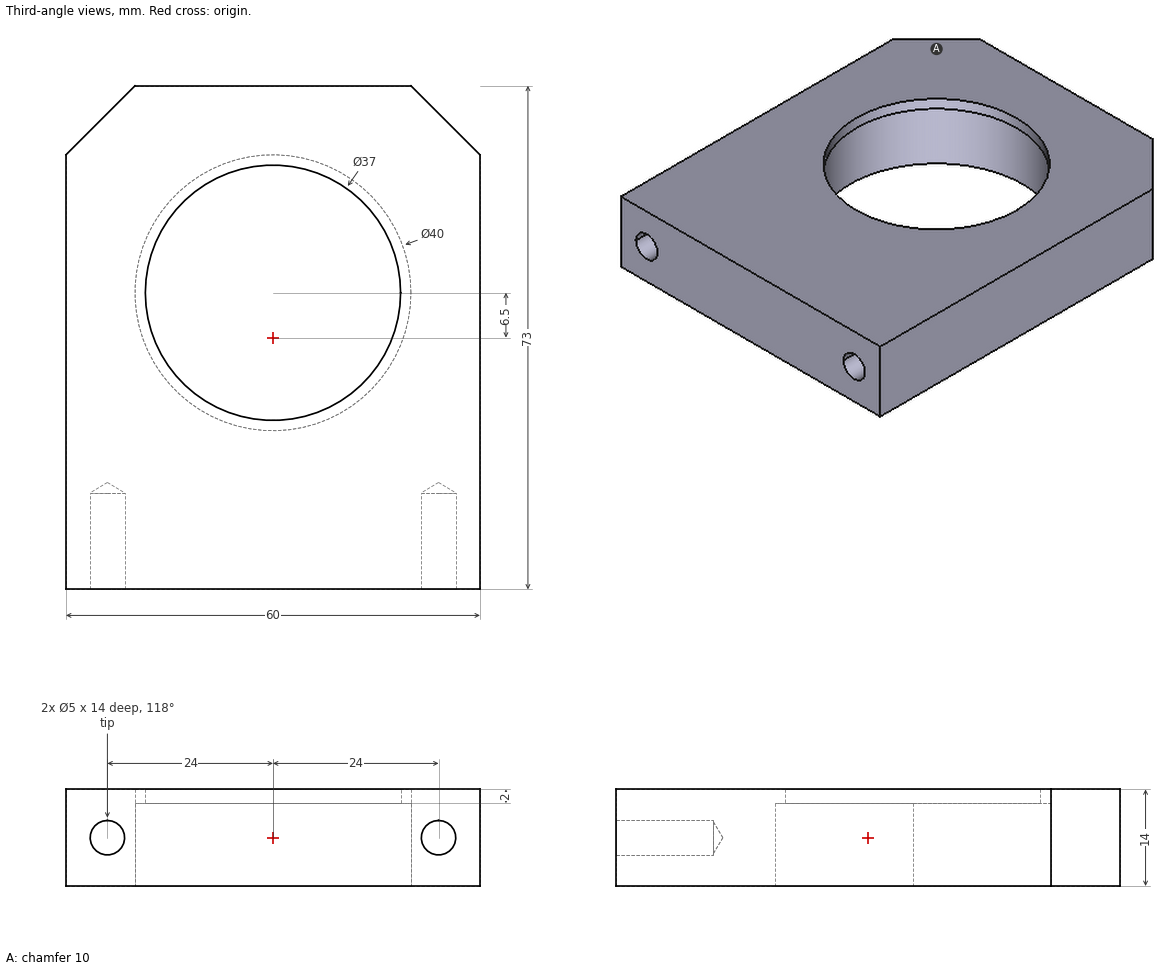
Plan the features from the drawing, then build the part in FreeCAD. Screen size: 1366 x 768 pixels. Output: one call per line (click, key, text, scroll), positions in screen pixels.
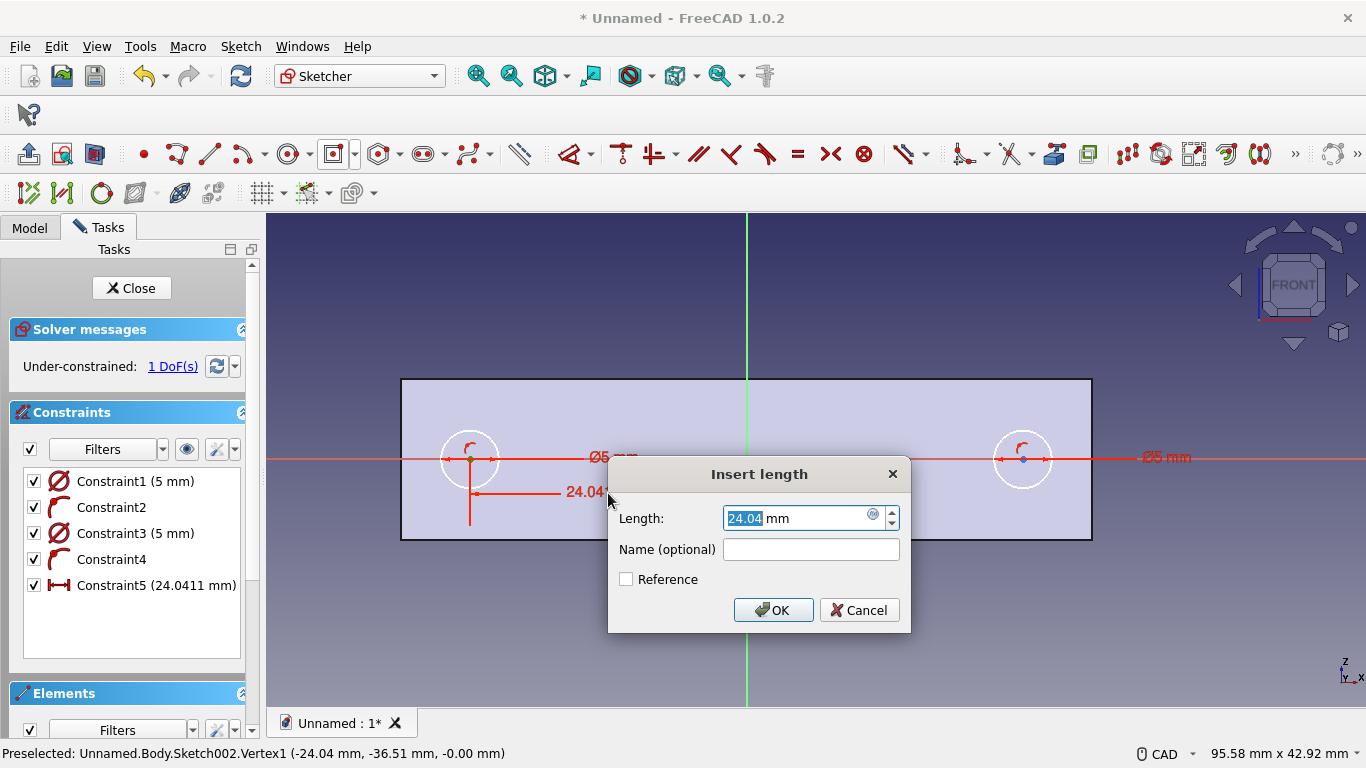
text(24)
key(Return)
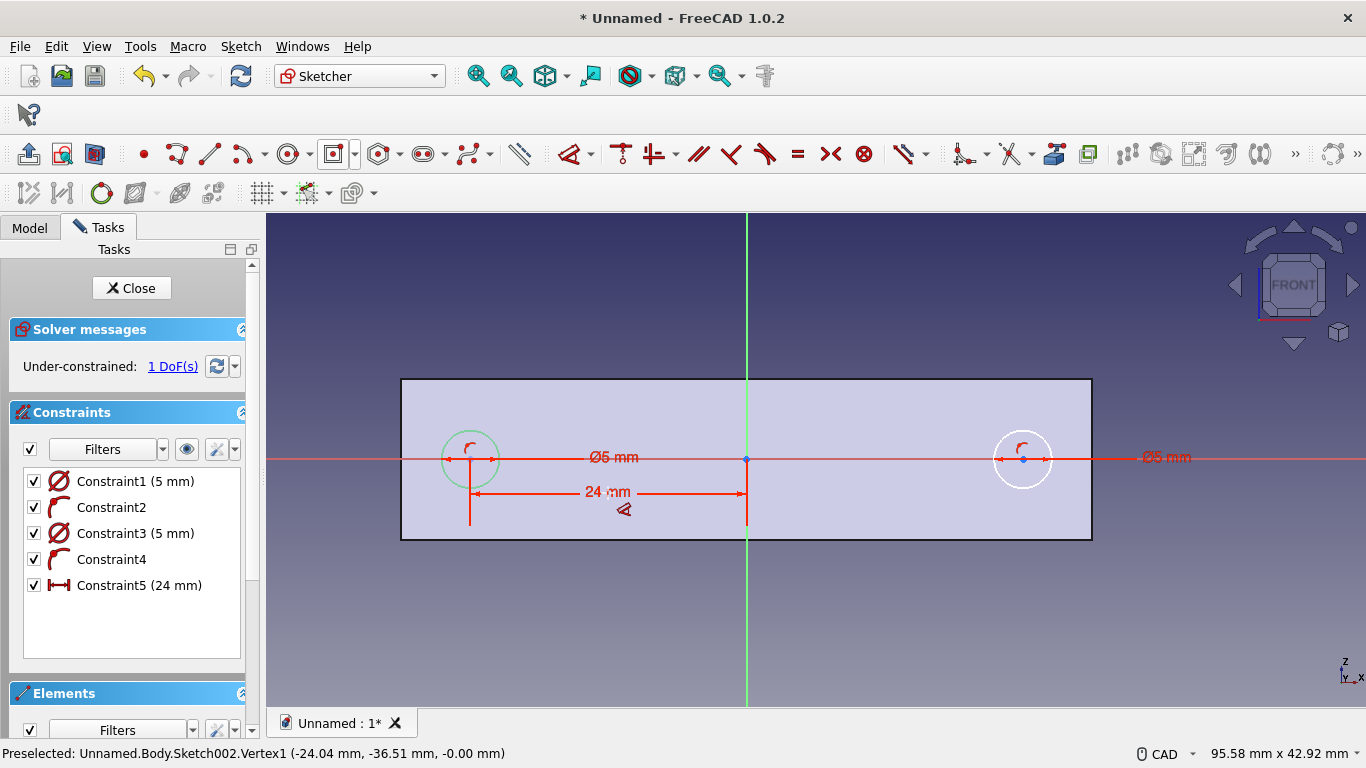
click(1023, 459)
click(885, 493)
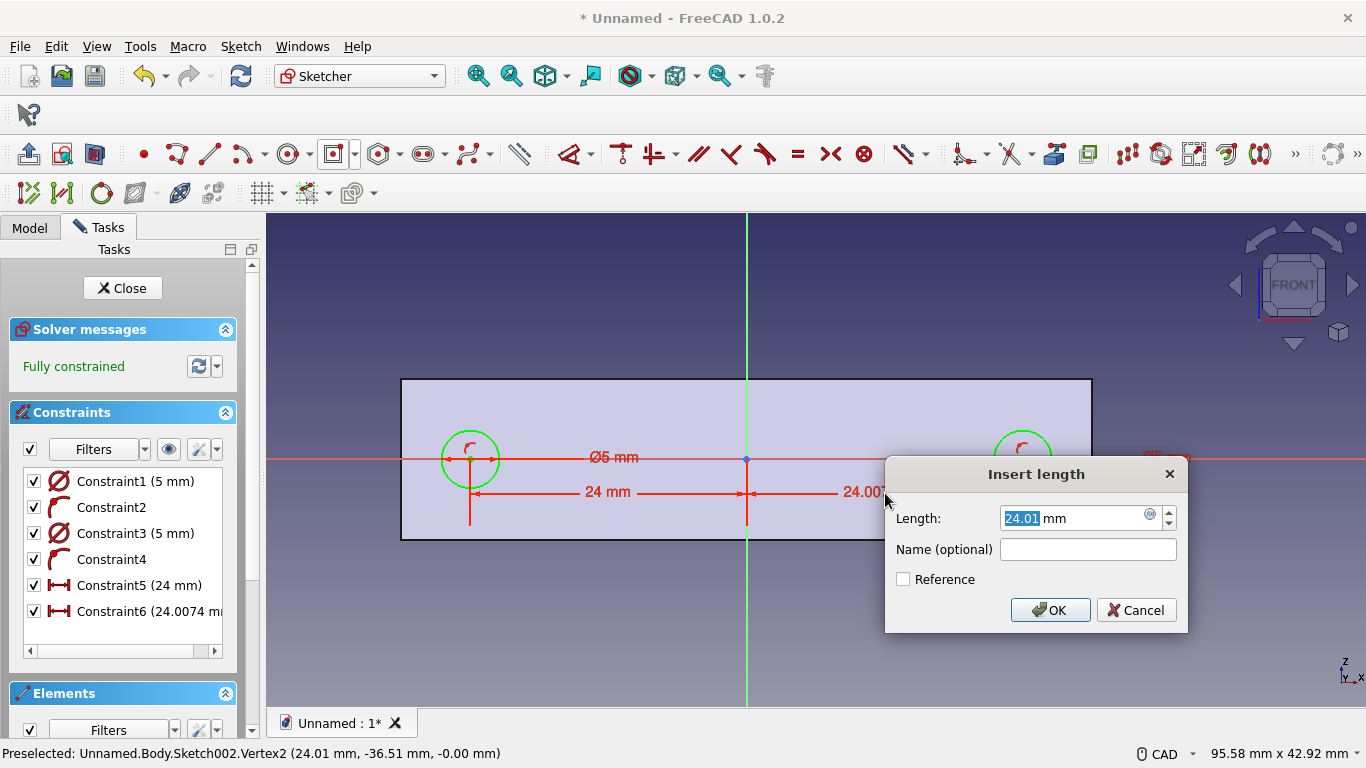
text(24)
key(Return)
key(Escape)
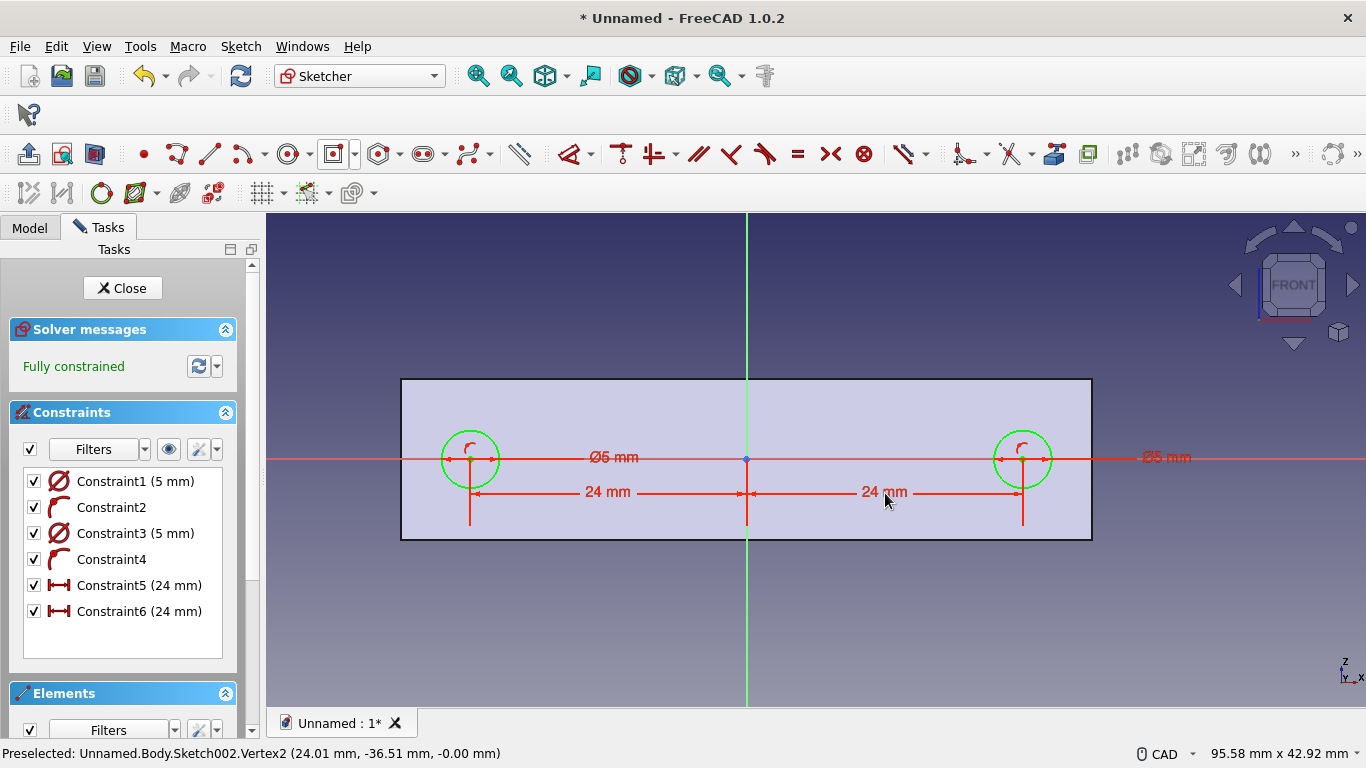
click(123, 288)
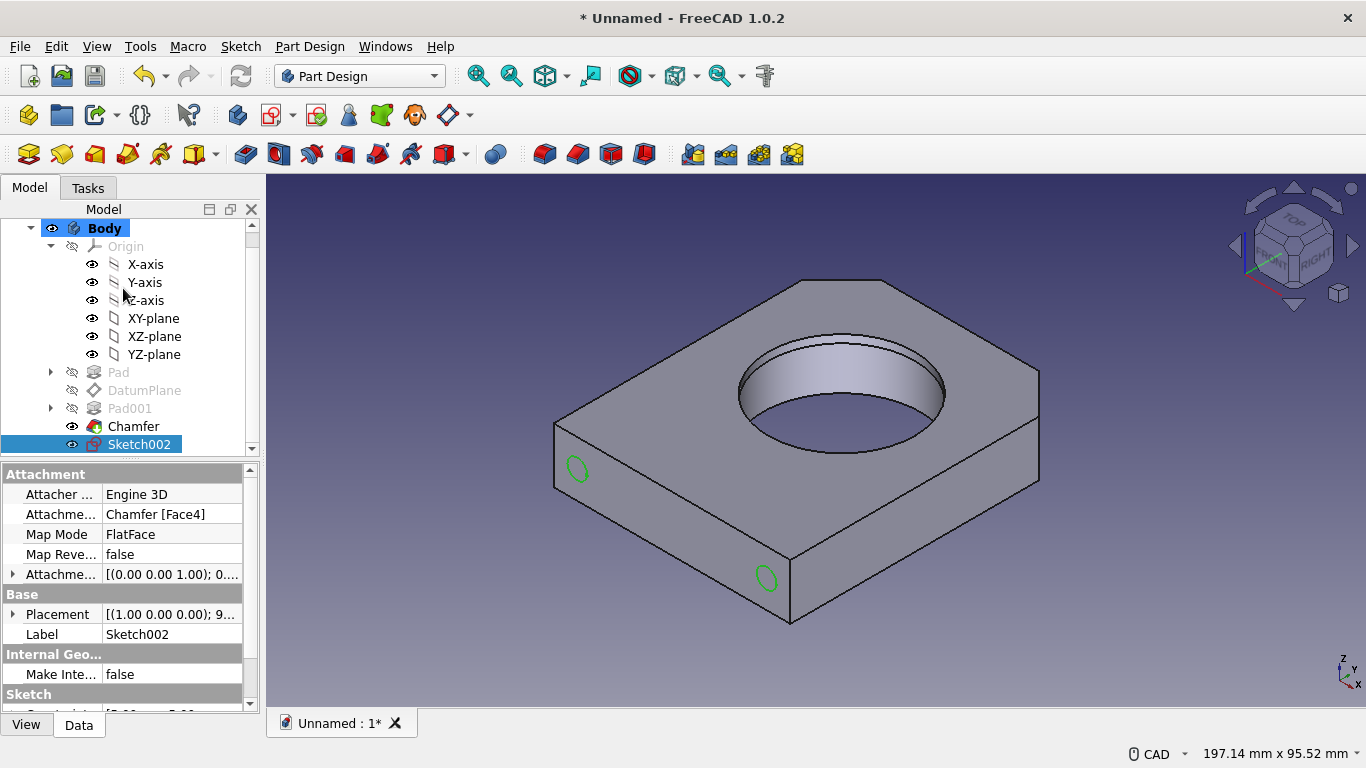
click(279, 154)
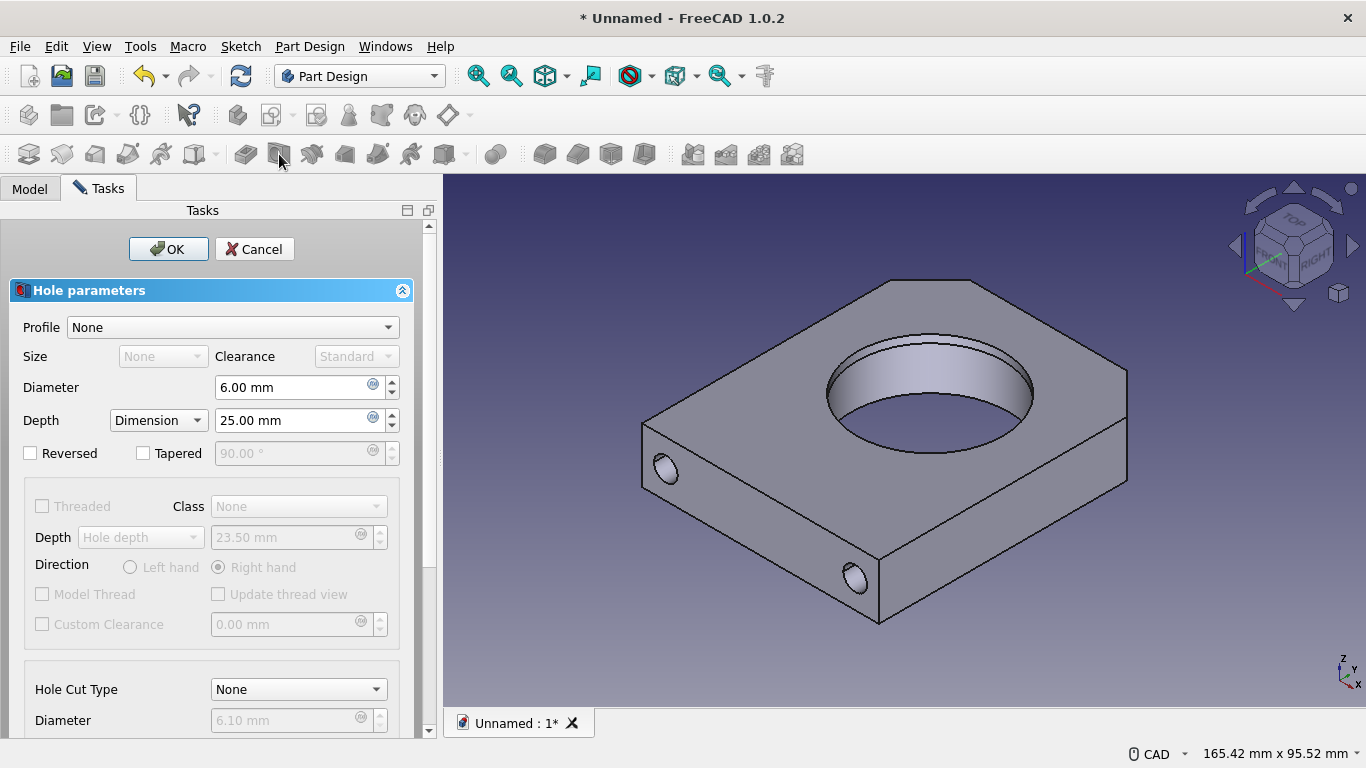
triple_click(300, 388)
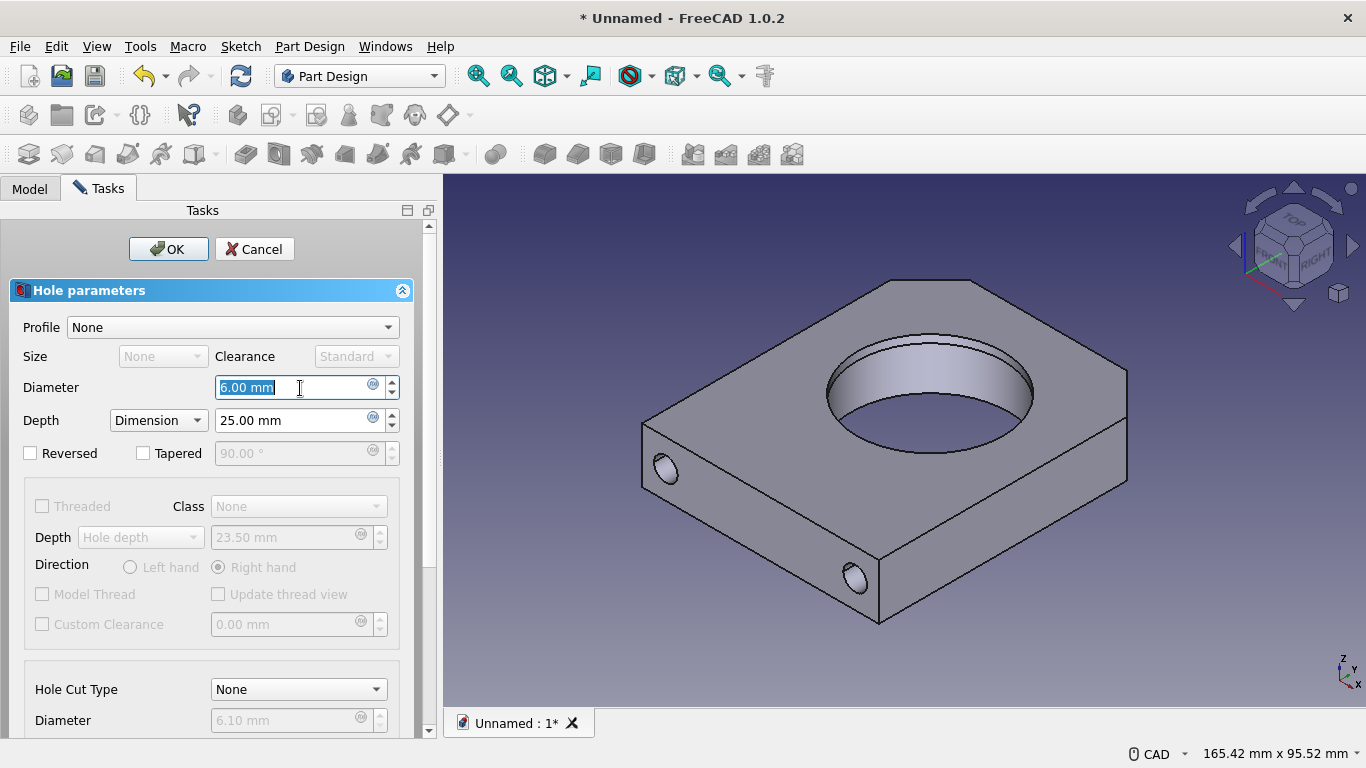
text(5)
key(Tab)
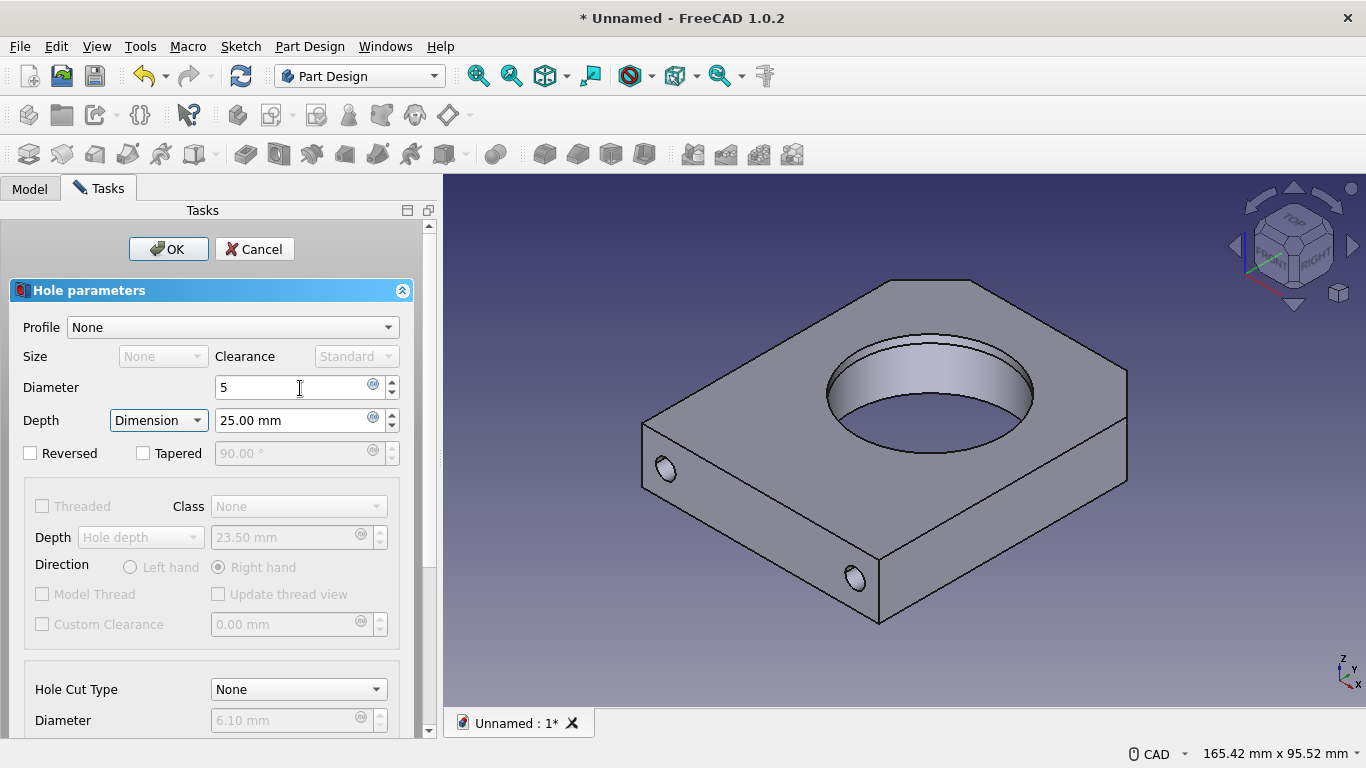
triple_click(300, 420)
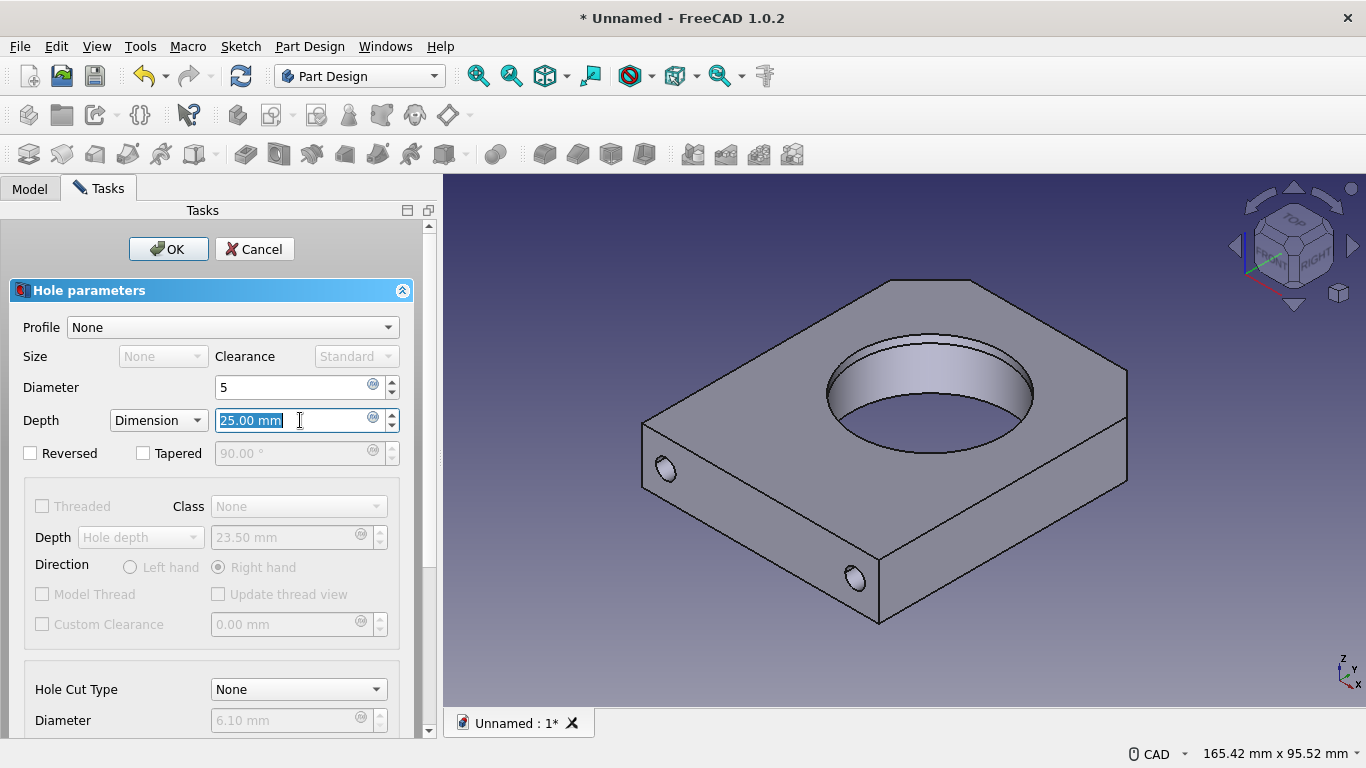
text(14)
key(Tab)